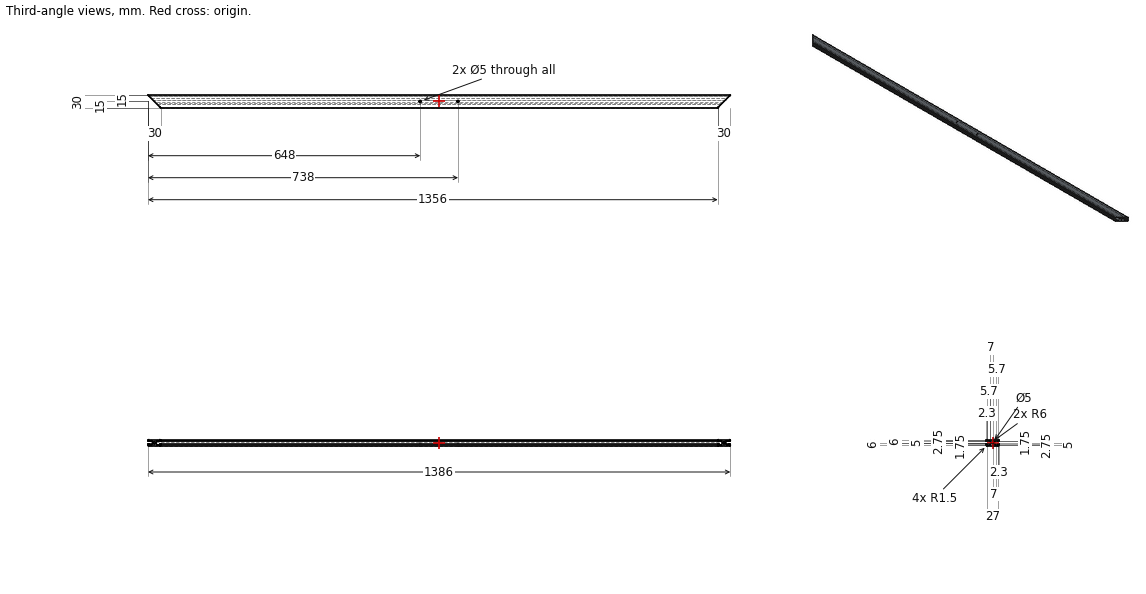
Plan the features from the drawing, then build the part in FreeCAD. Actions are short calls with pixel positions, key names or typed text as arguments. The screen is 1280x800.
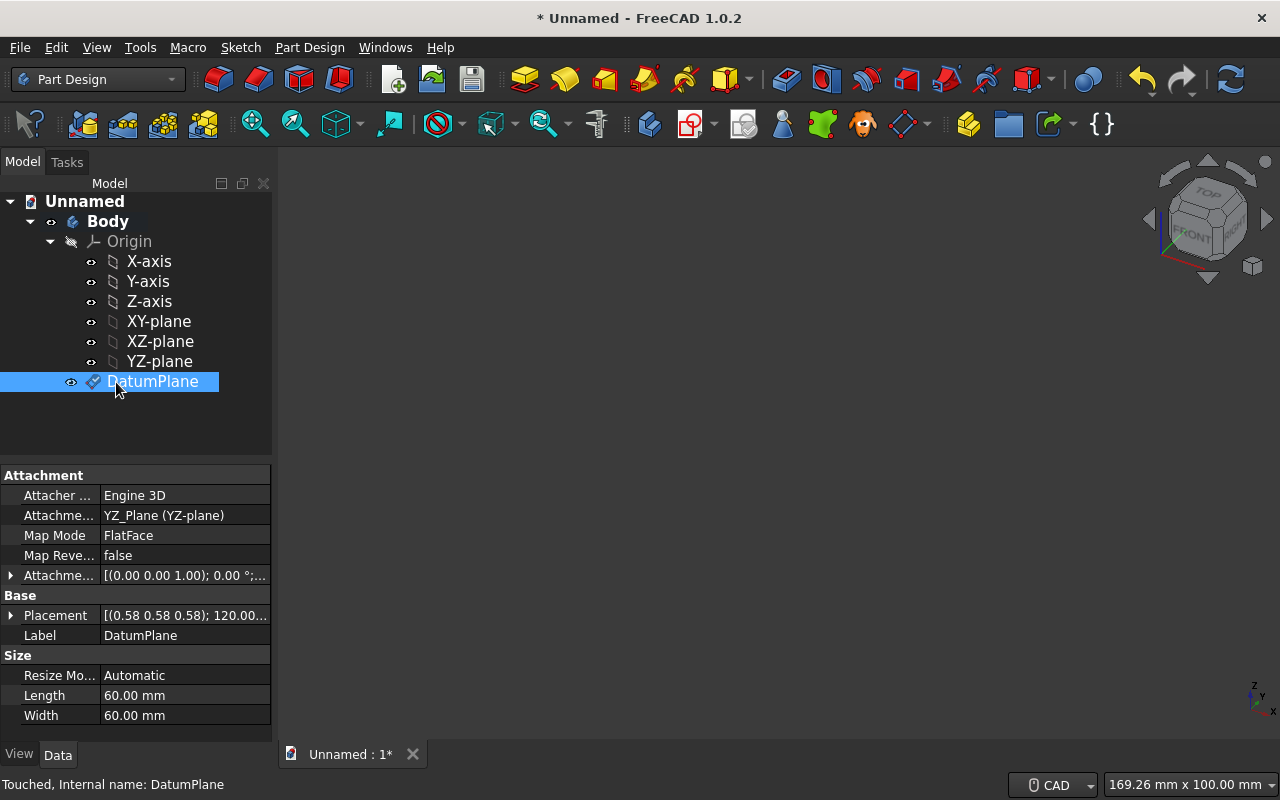
click(690, 124)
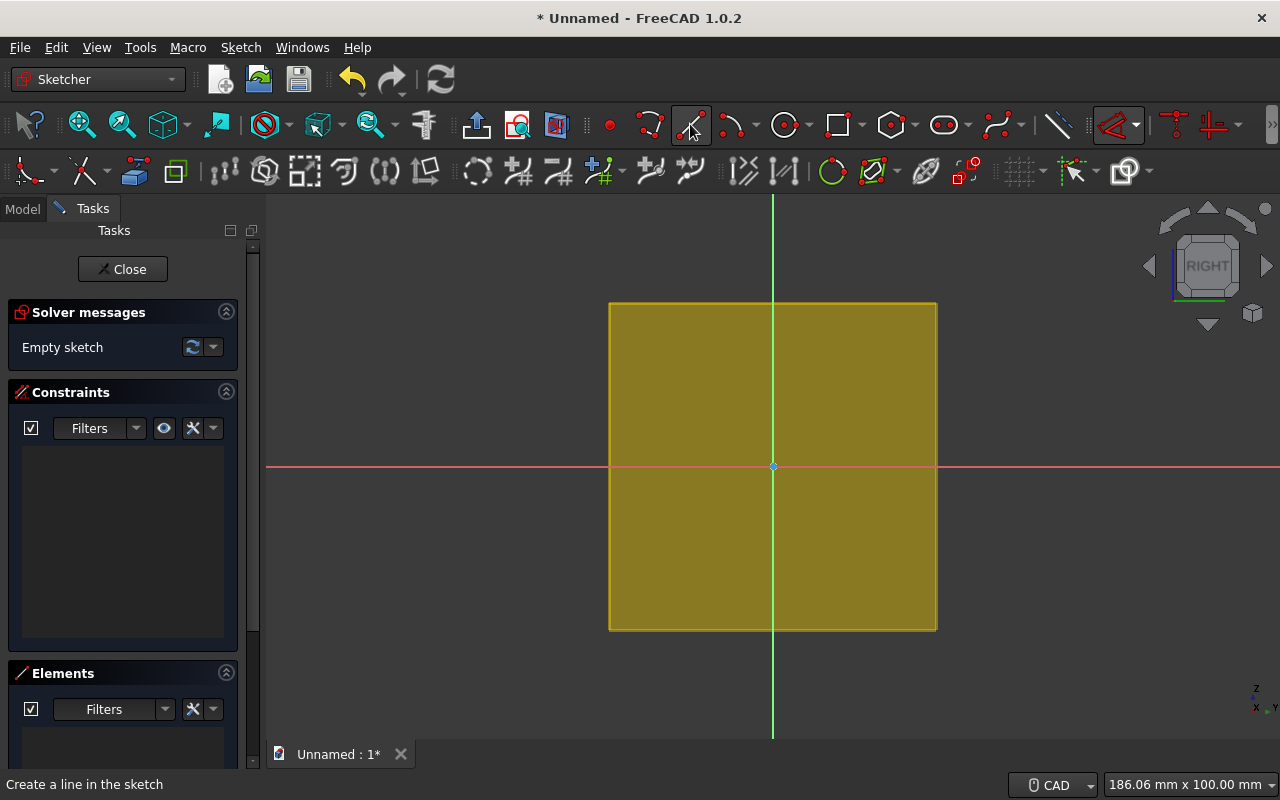
scroll(803, 466, up, 6)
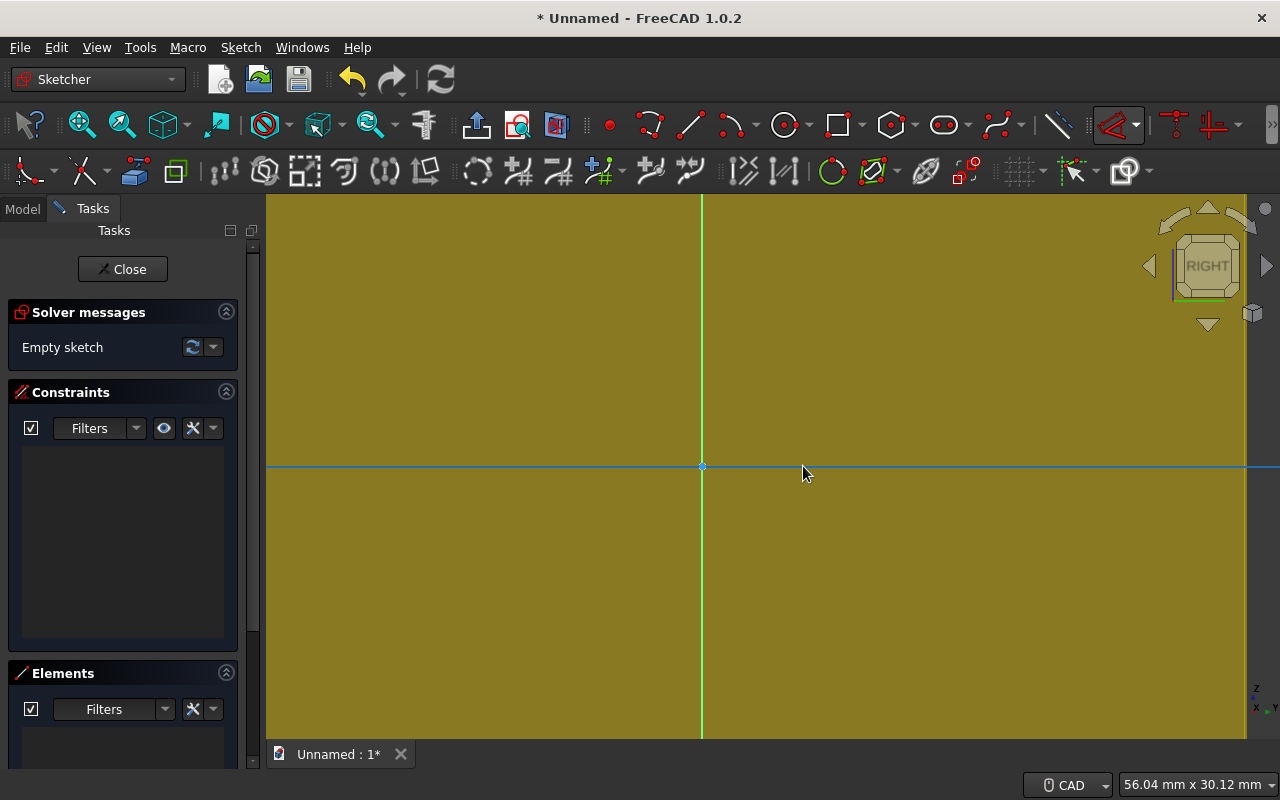
key(g)
key(m)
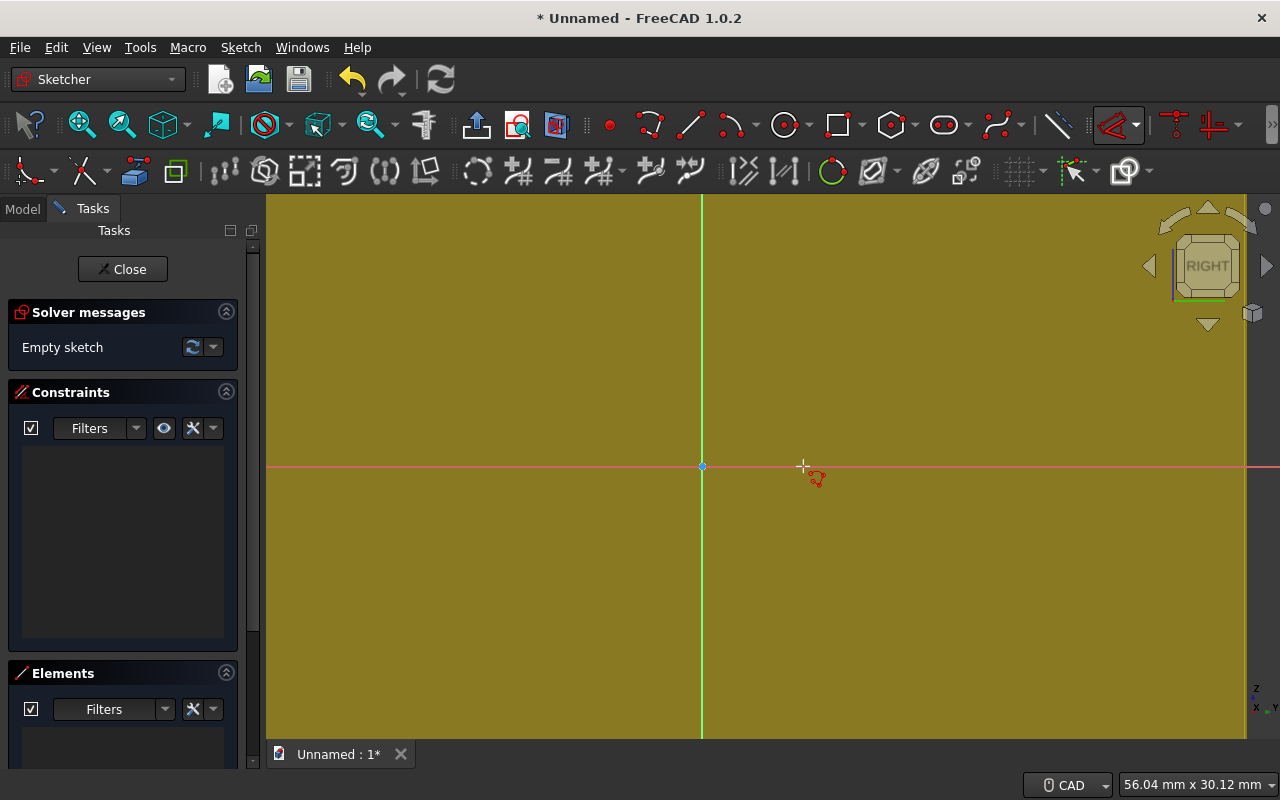
click(431, 358)
click(431, 408)
click(472, 408)
click(472, 376)
click(576, 376)
right_click(576, 376)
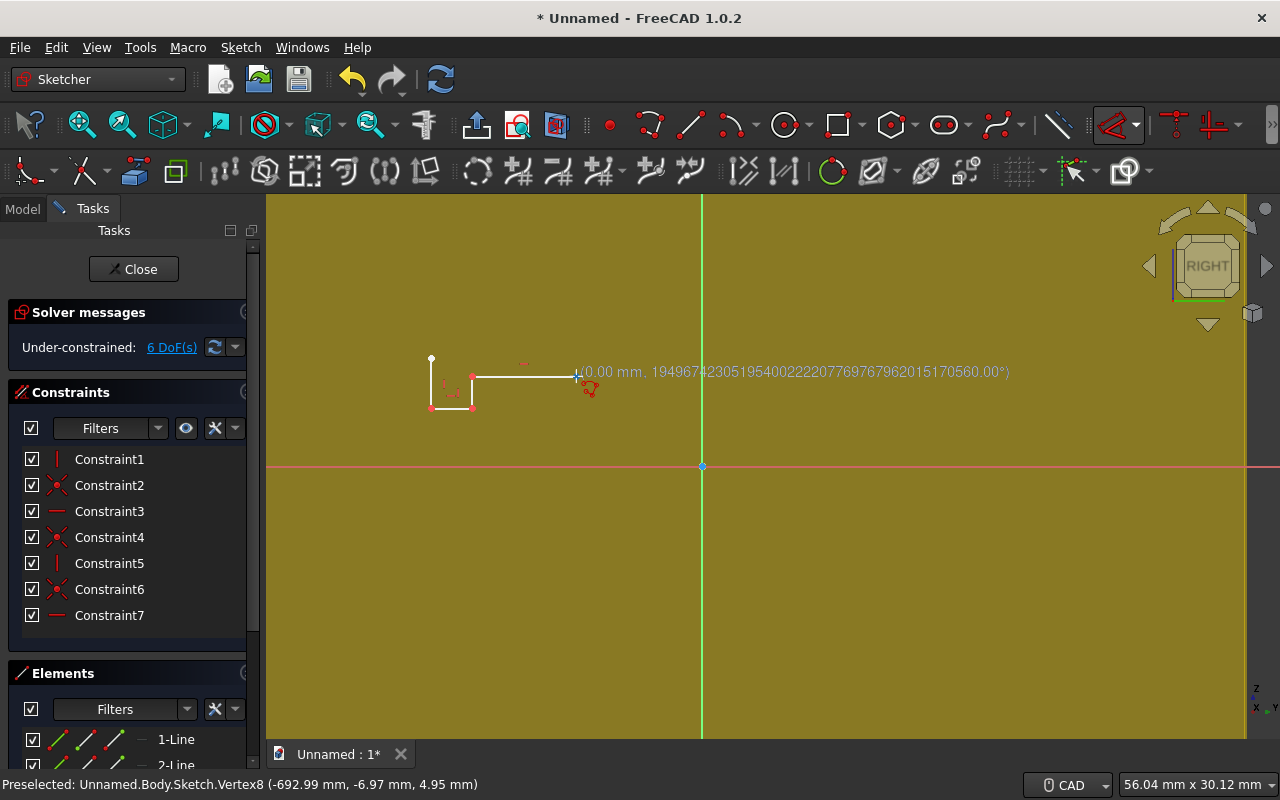
click(576, 557)
click(472, 557)
click(472, 525)
click(431, 525)
click(431, 575)
right_click(431, 575)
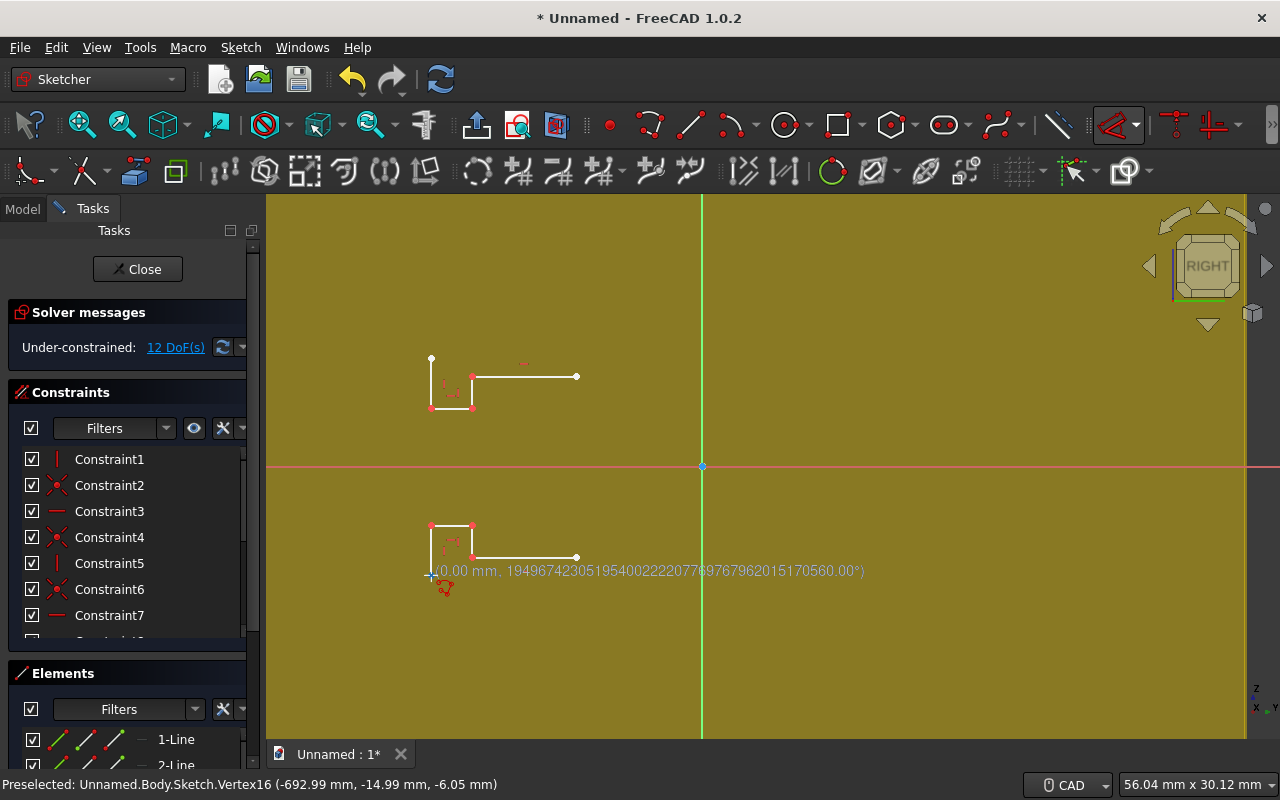
key(g)
key(l)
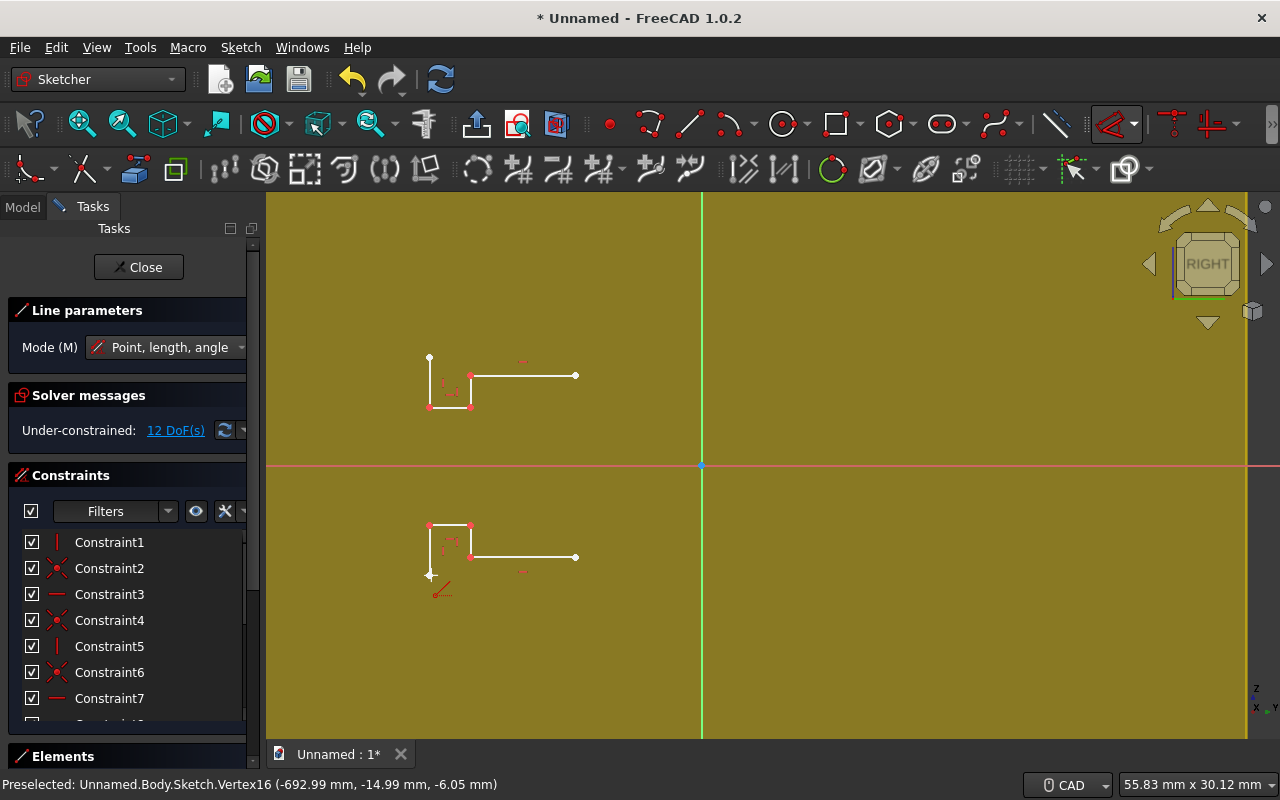
click(457, 602)
click(947, 602)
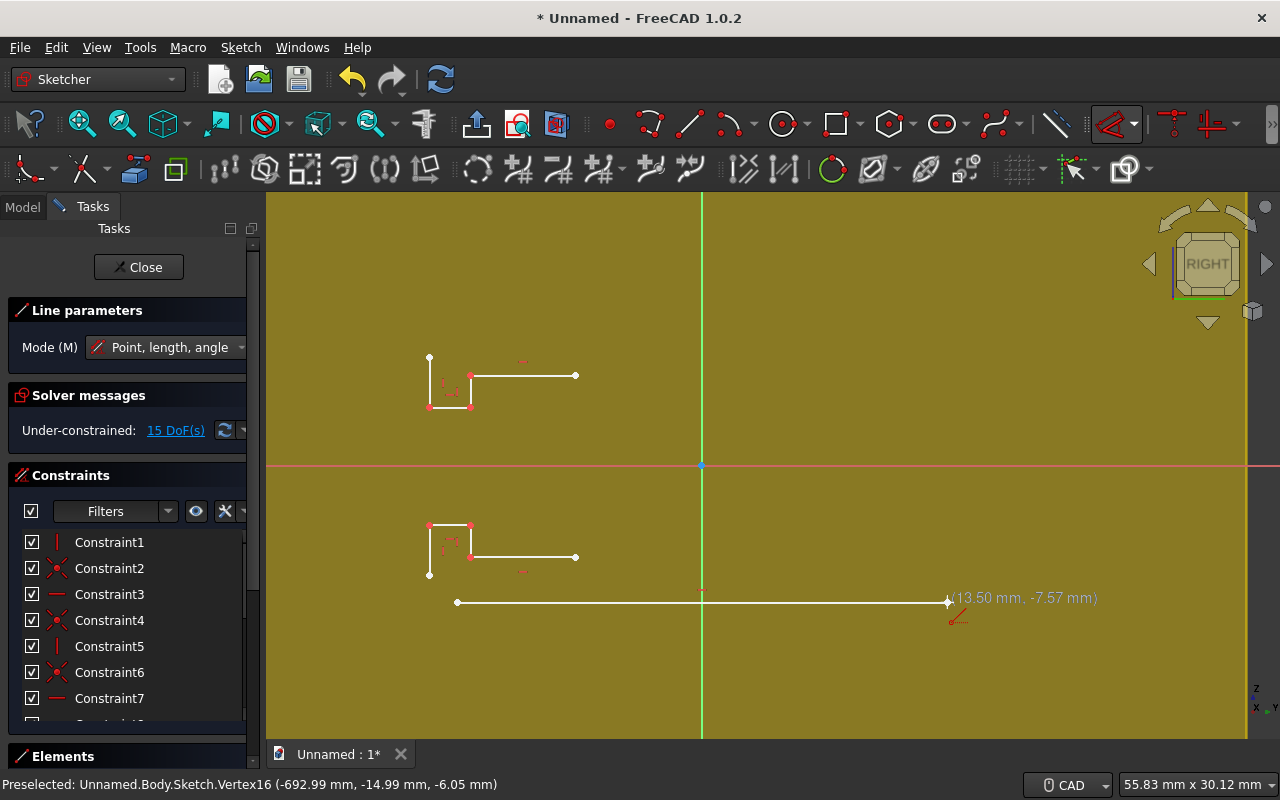
click(650, 124)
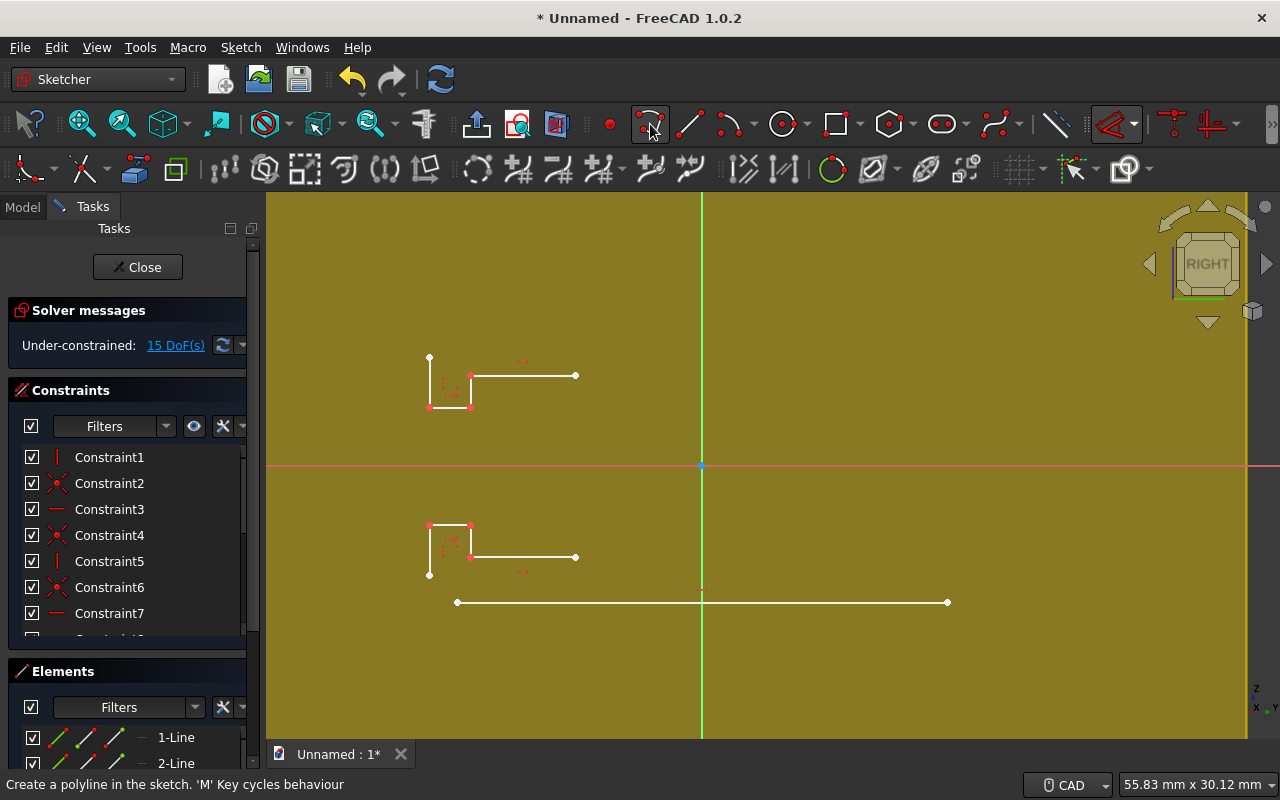
click(974, 574)
click(974, 525)
click(933, 525)
click(933, 556)
click(829, 556)
right_click(829, 556)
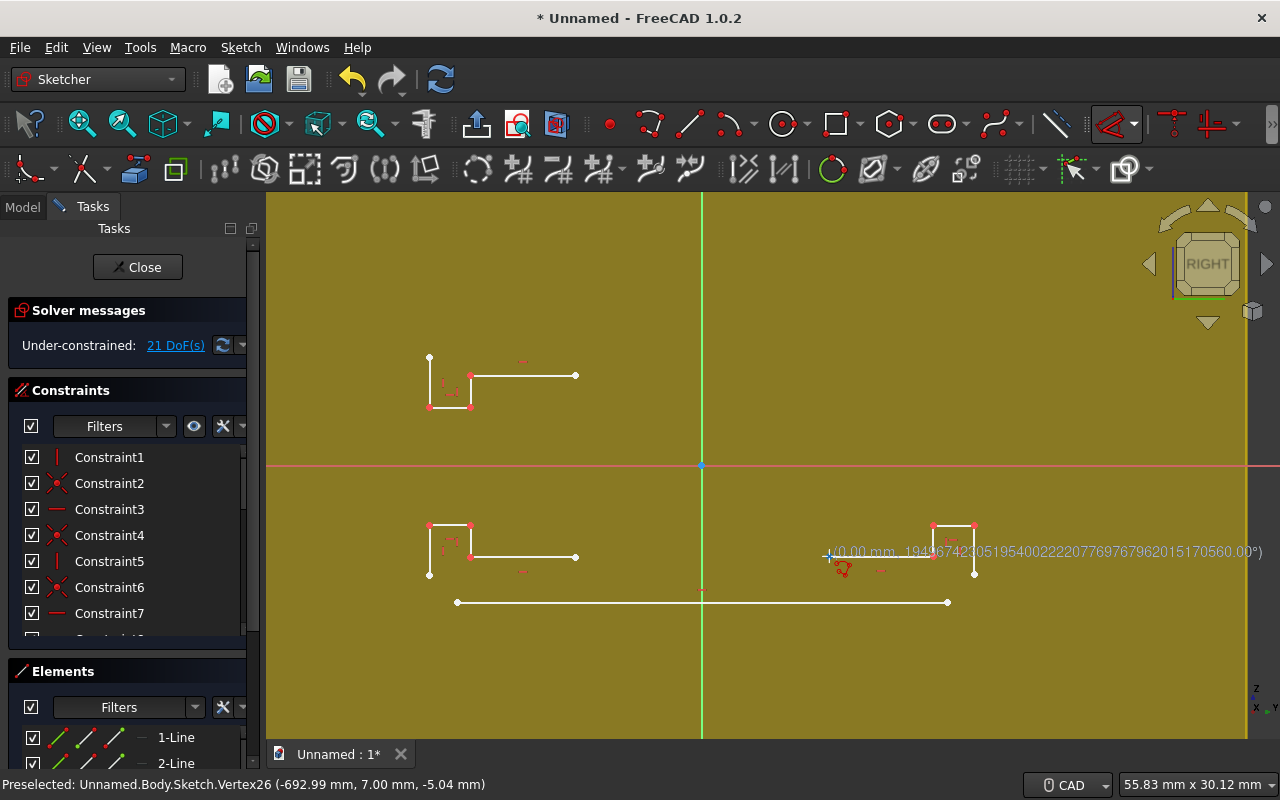
click(829, 375)
click(933, 375)
click(933, 406)
click(974, 406)
click(974, 357)
right_click(974, 357)